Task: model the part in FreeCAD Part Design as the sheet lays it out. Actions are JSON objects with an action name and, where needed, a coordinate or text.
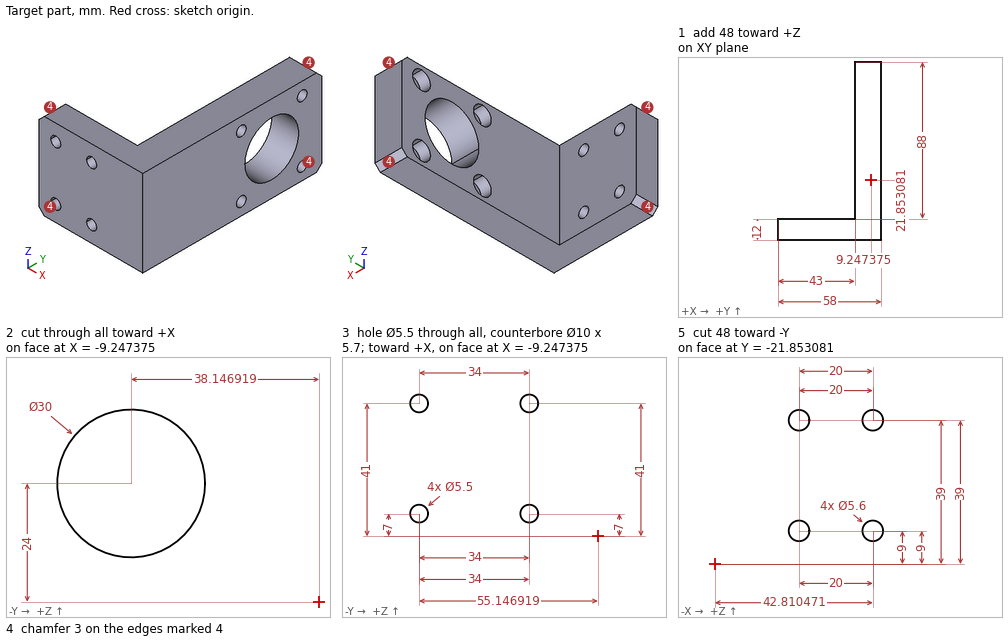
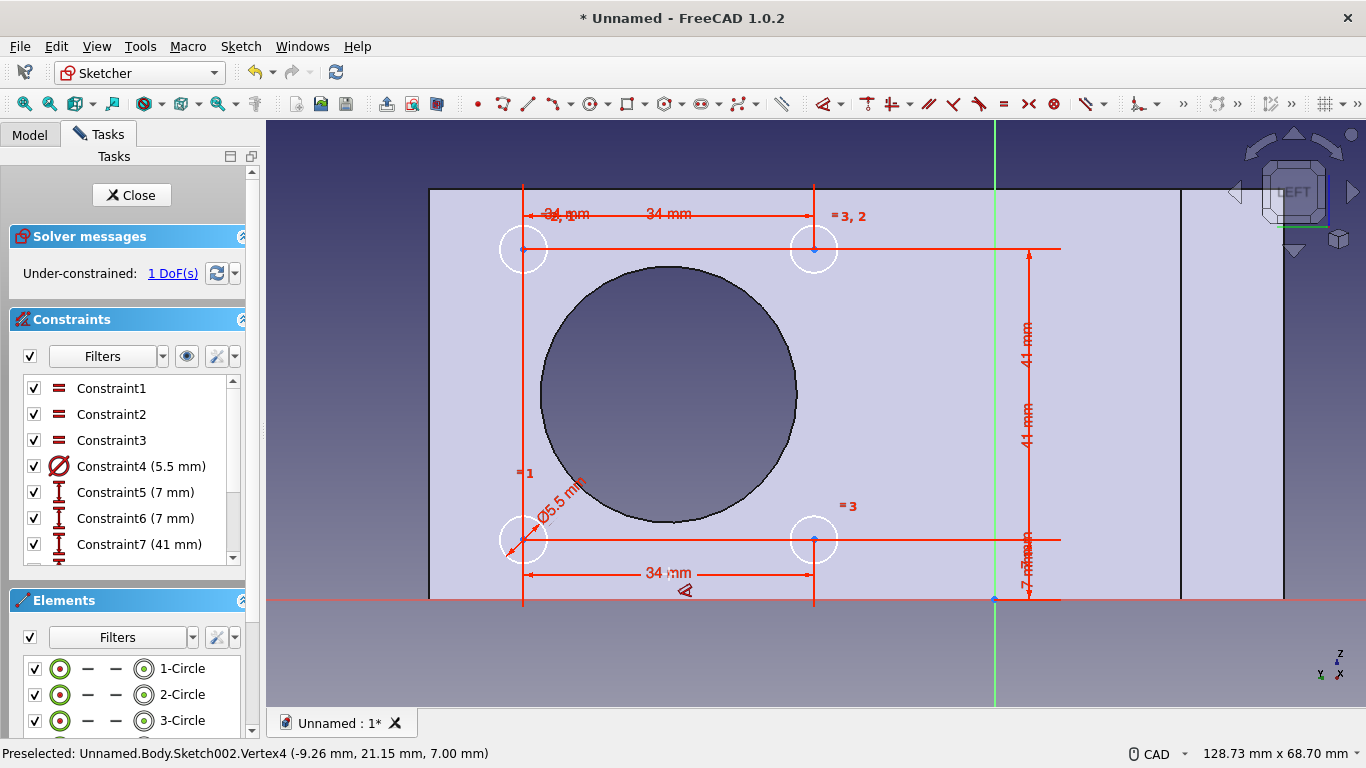
{"action": "left_click", "coordinate": [523, 540]}
{"action": "left_click", "coordinate": [759, 634]}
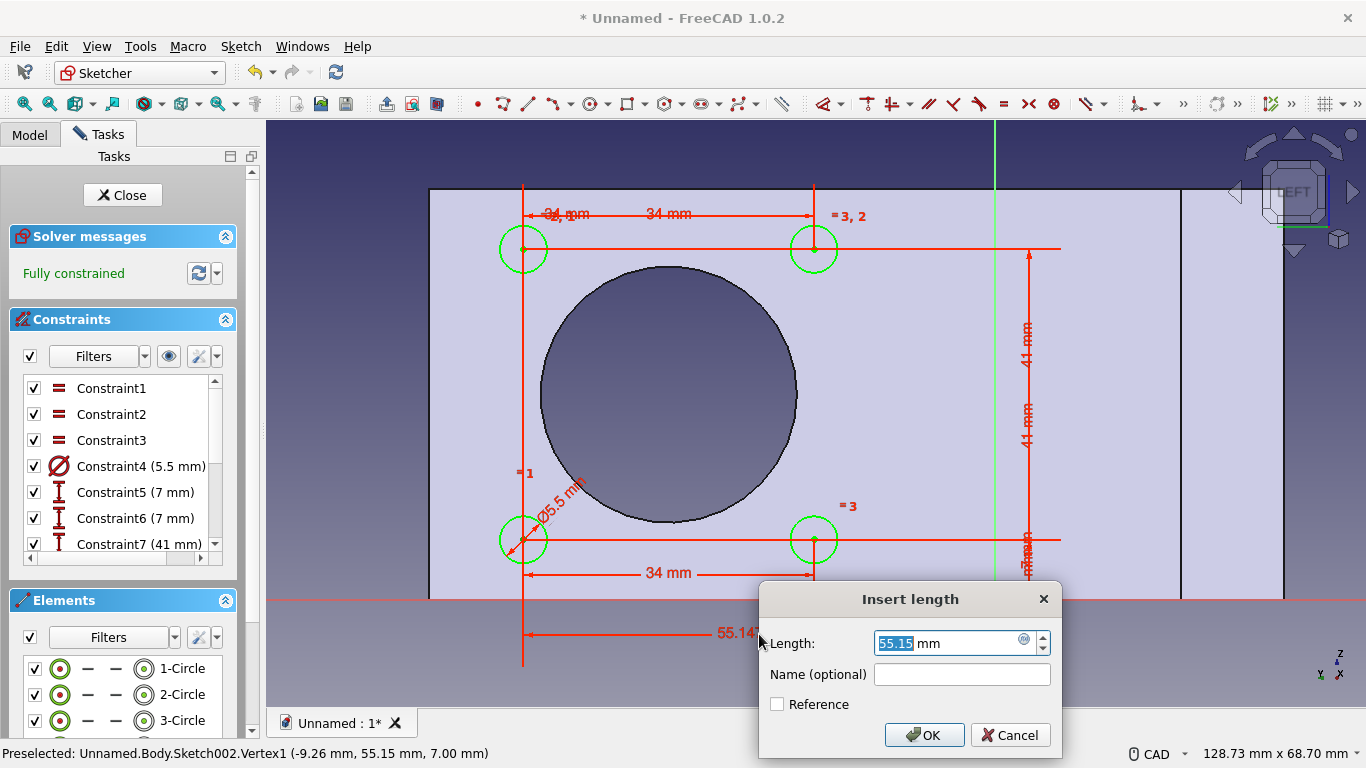
{"action": "type", "text": "55.146919"}
{"action": "key", "text": "Return"}
{"action": "key", "text": "Escape"}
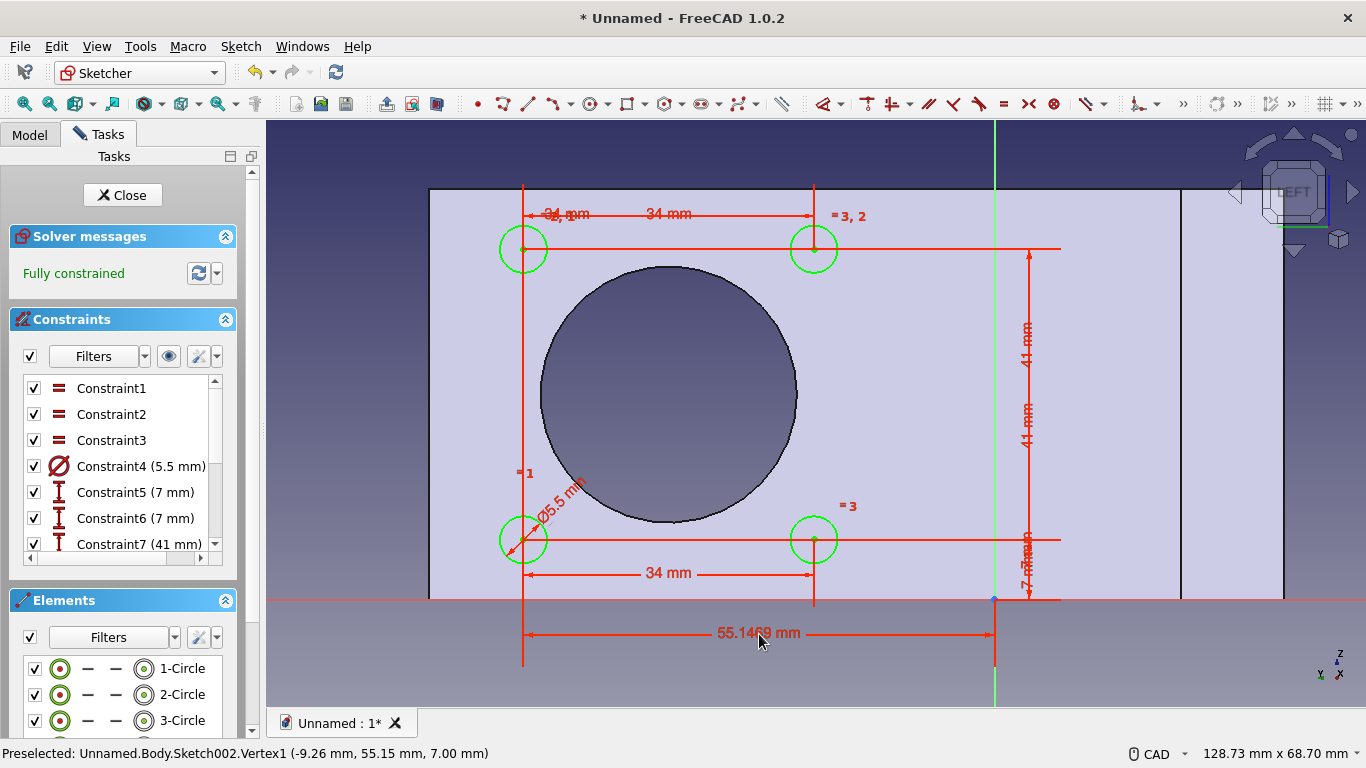
{"action": "left_click", "coordinate": [123, 195]}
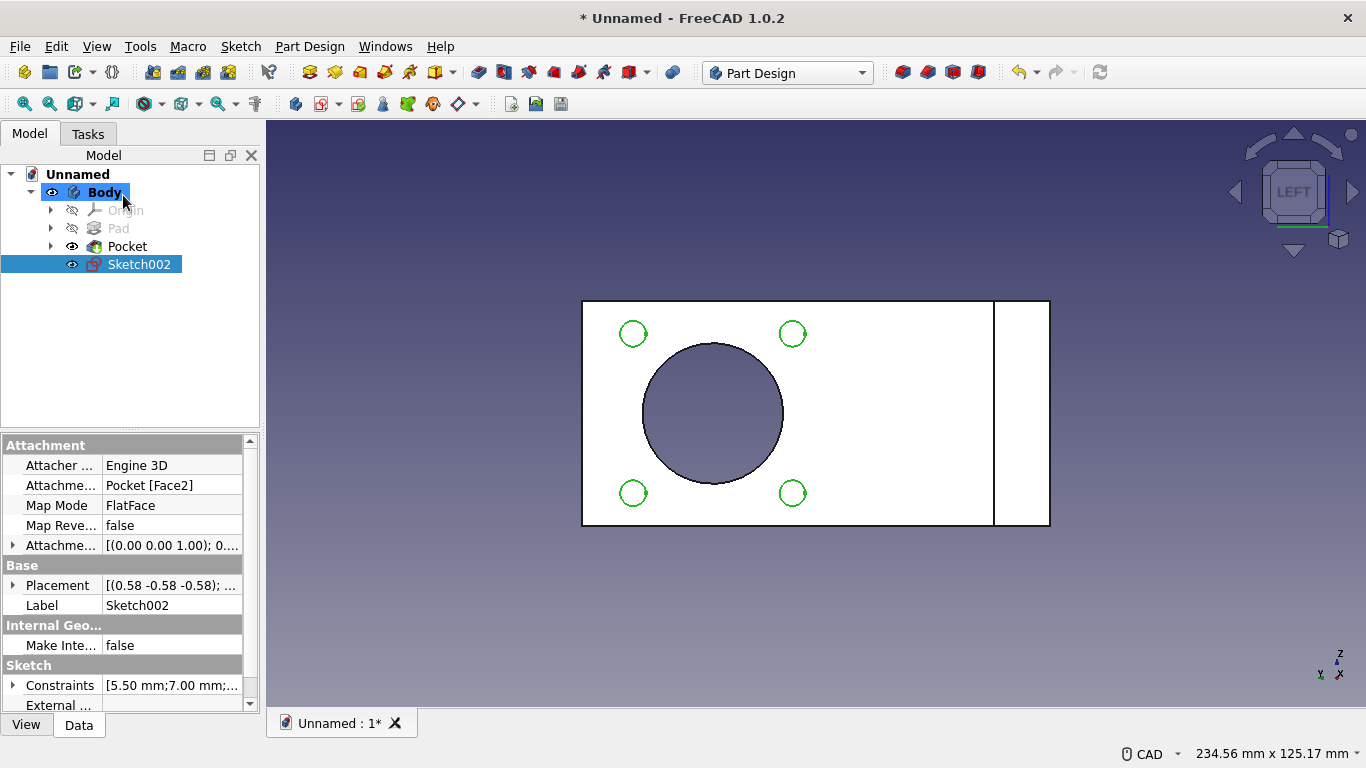
{"action": "left_click", "coordinate": [504, 72]}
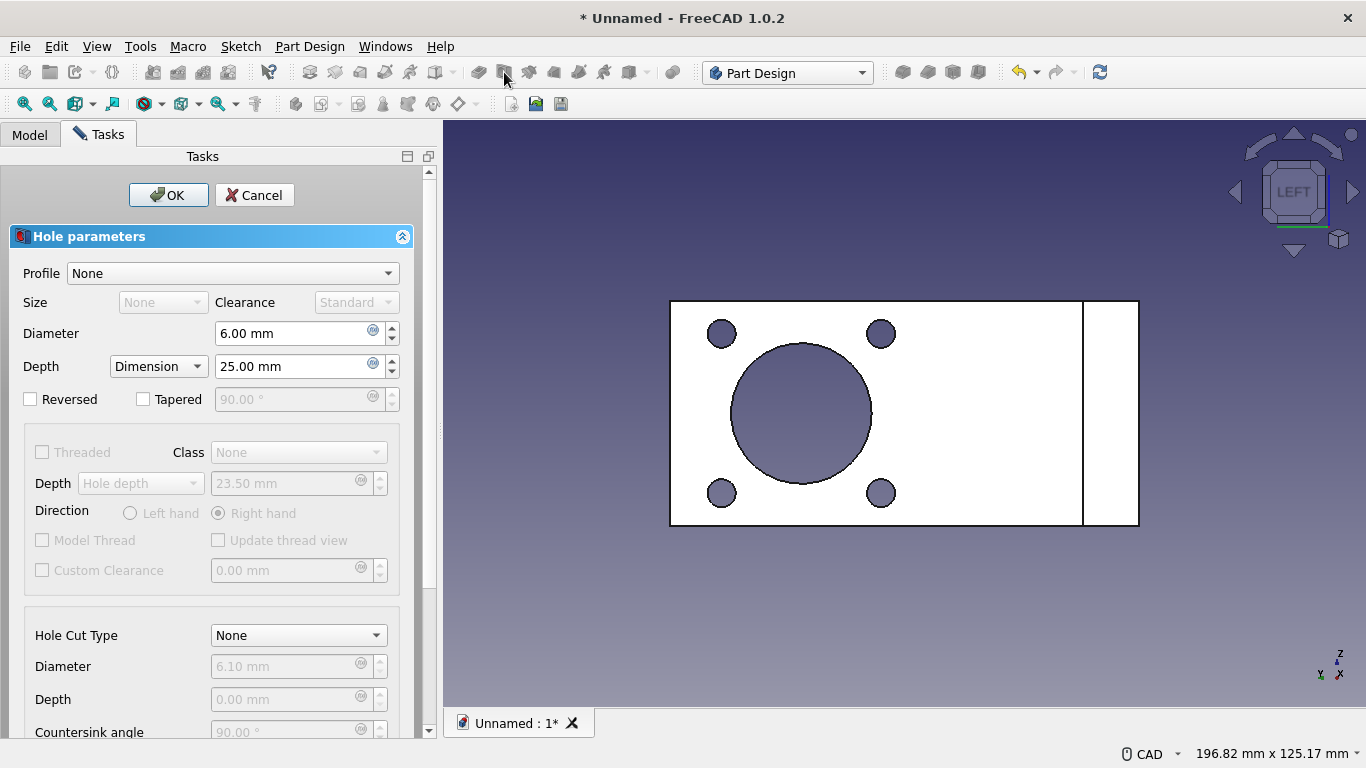
{"action": "triple_click", "coordinate": [300, 334]}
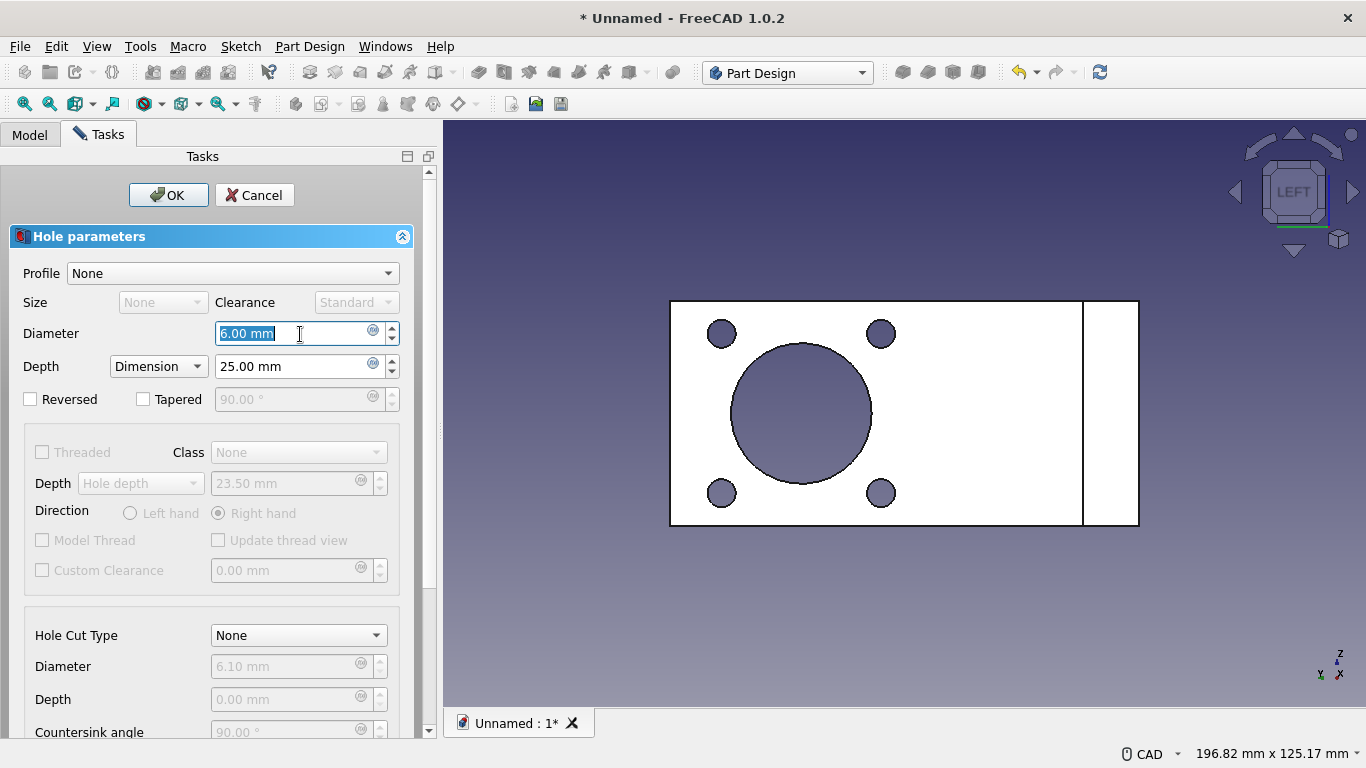
{"action": "type", "text": "5.5"}
{"action": "key", "text": "Tab"}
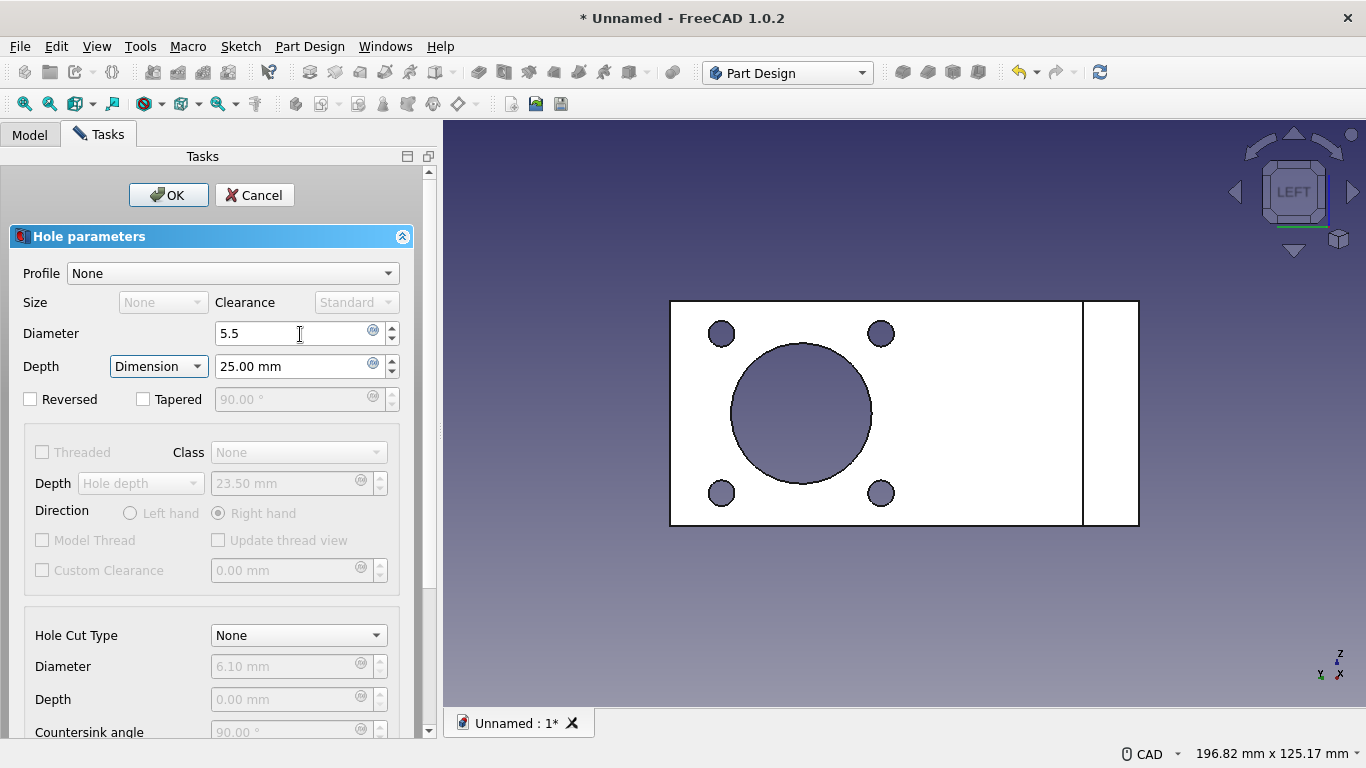
{"action": "left_click", "coordinate": [160, 366]}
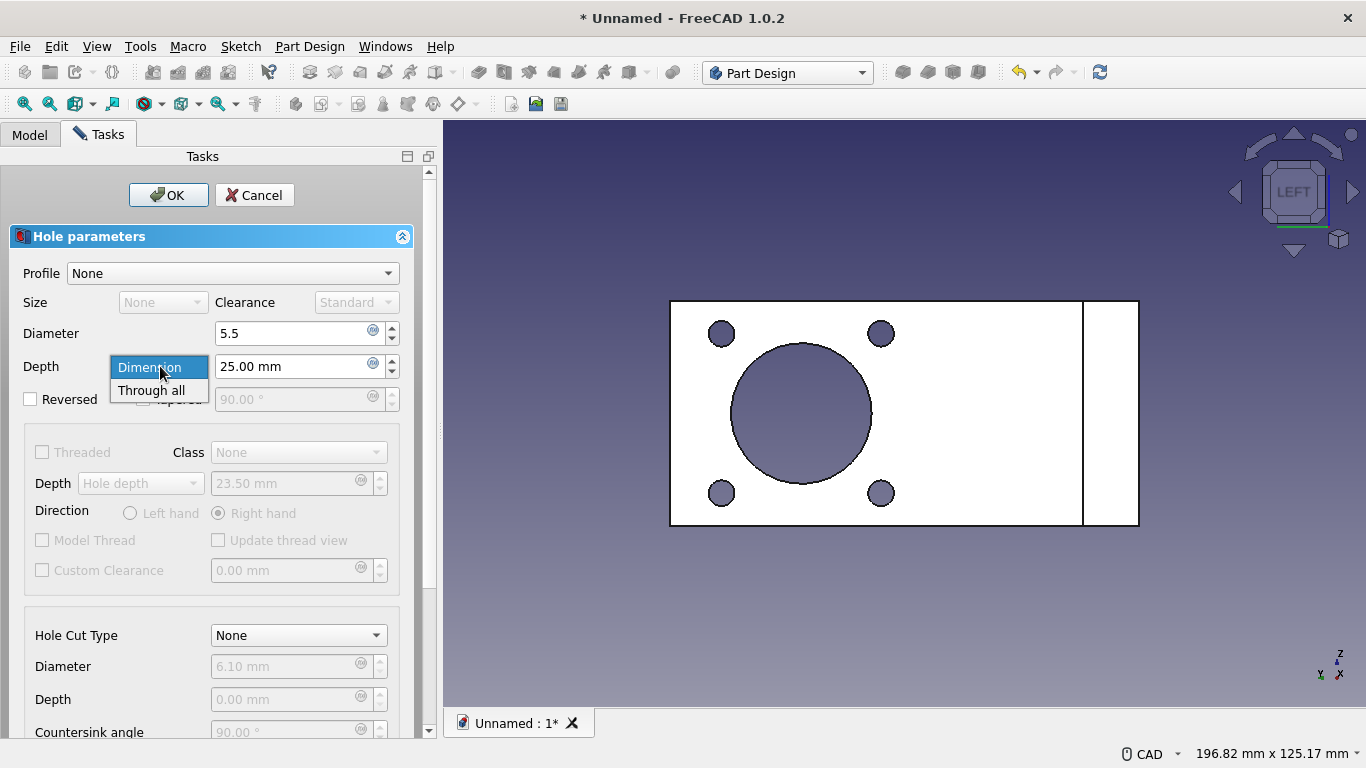
{"action": "left_click", "coordinate": [158, 390]}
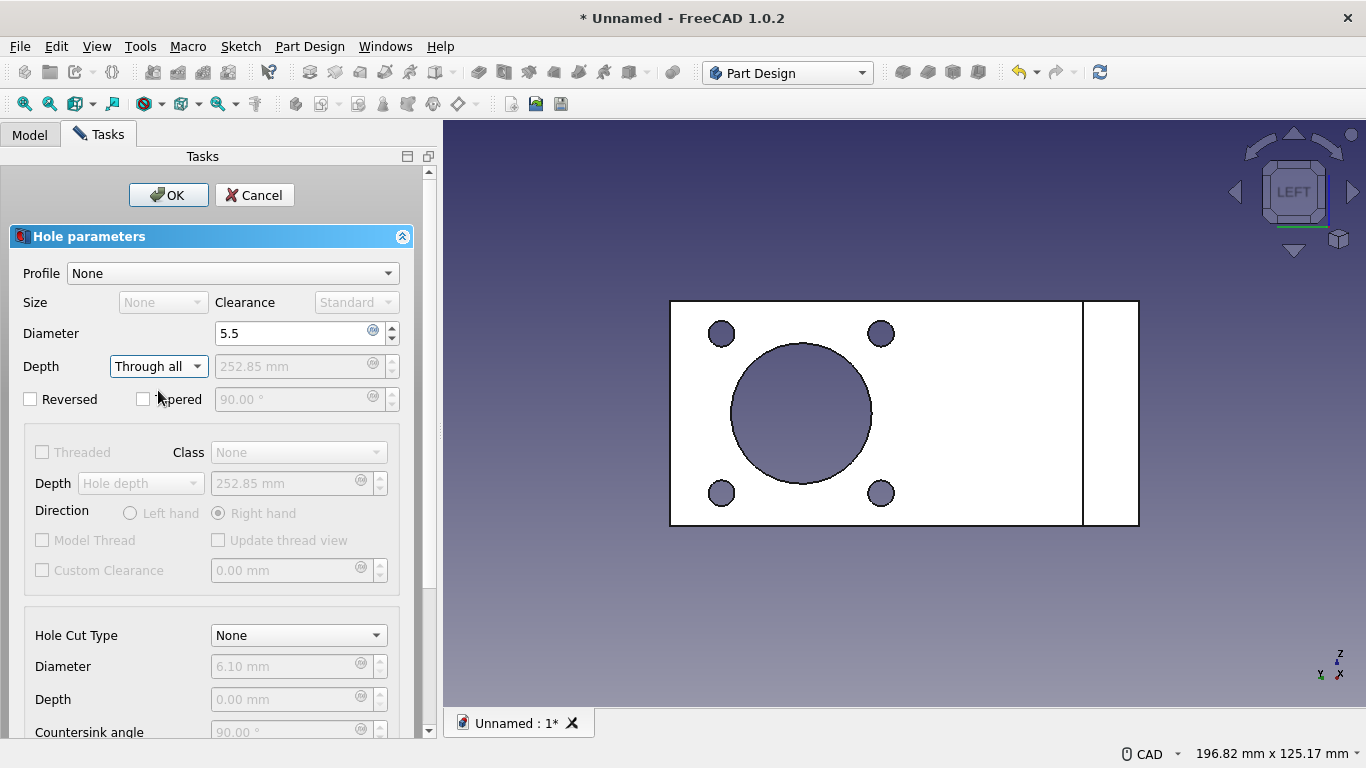
{"action": "left_click", "coordinate": [300, 636]}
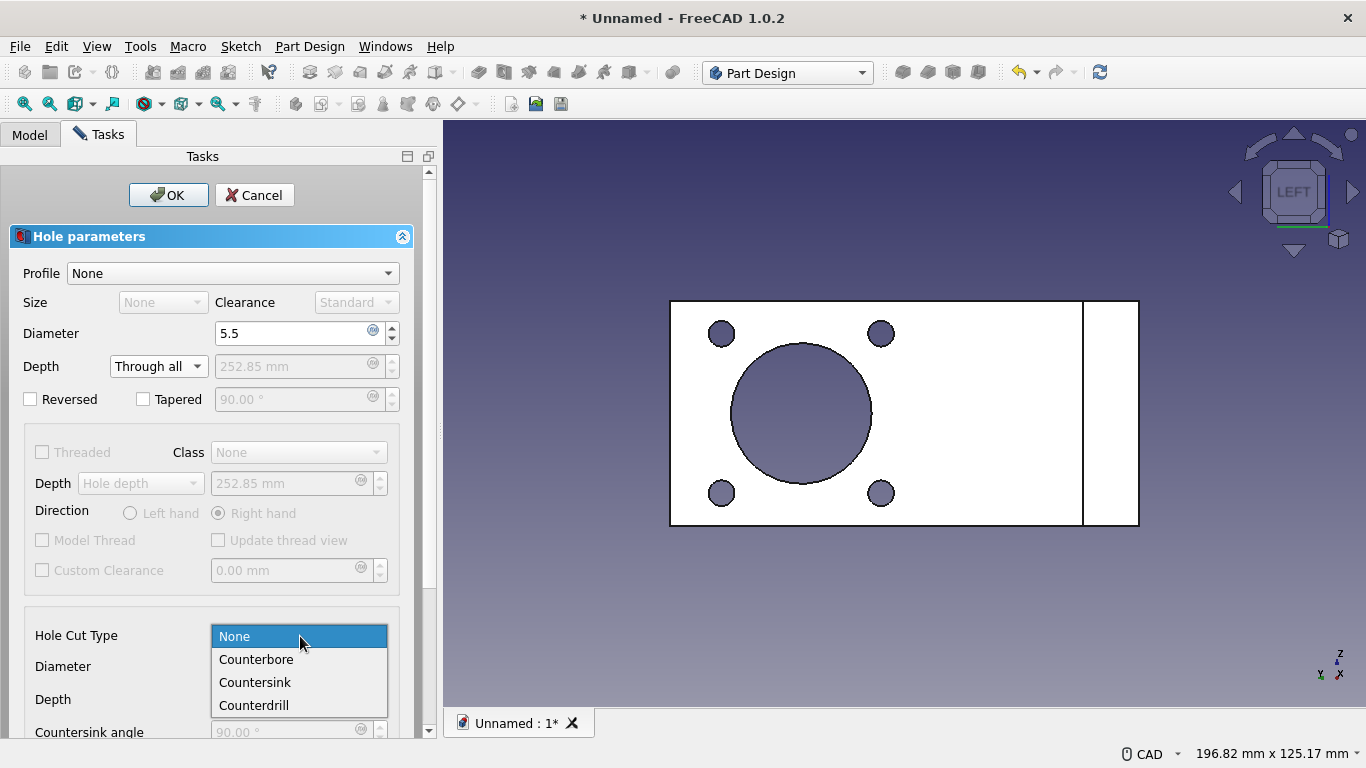
{"action": "left_click", "coordinate": [298, 660]}